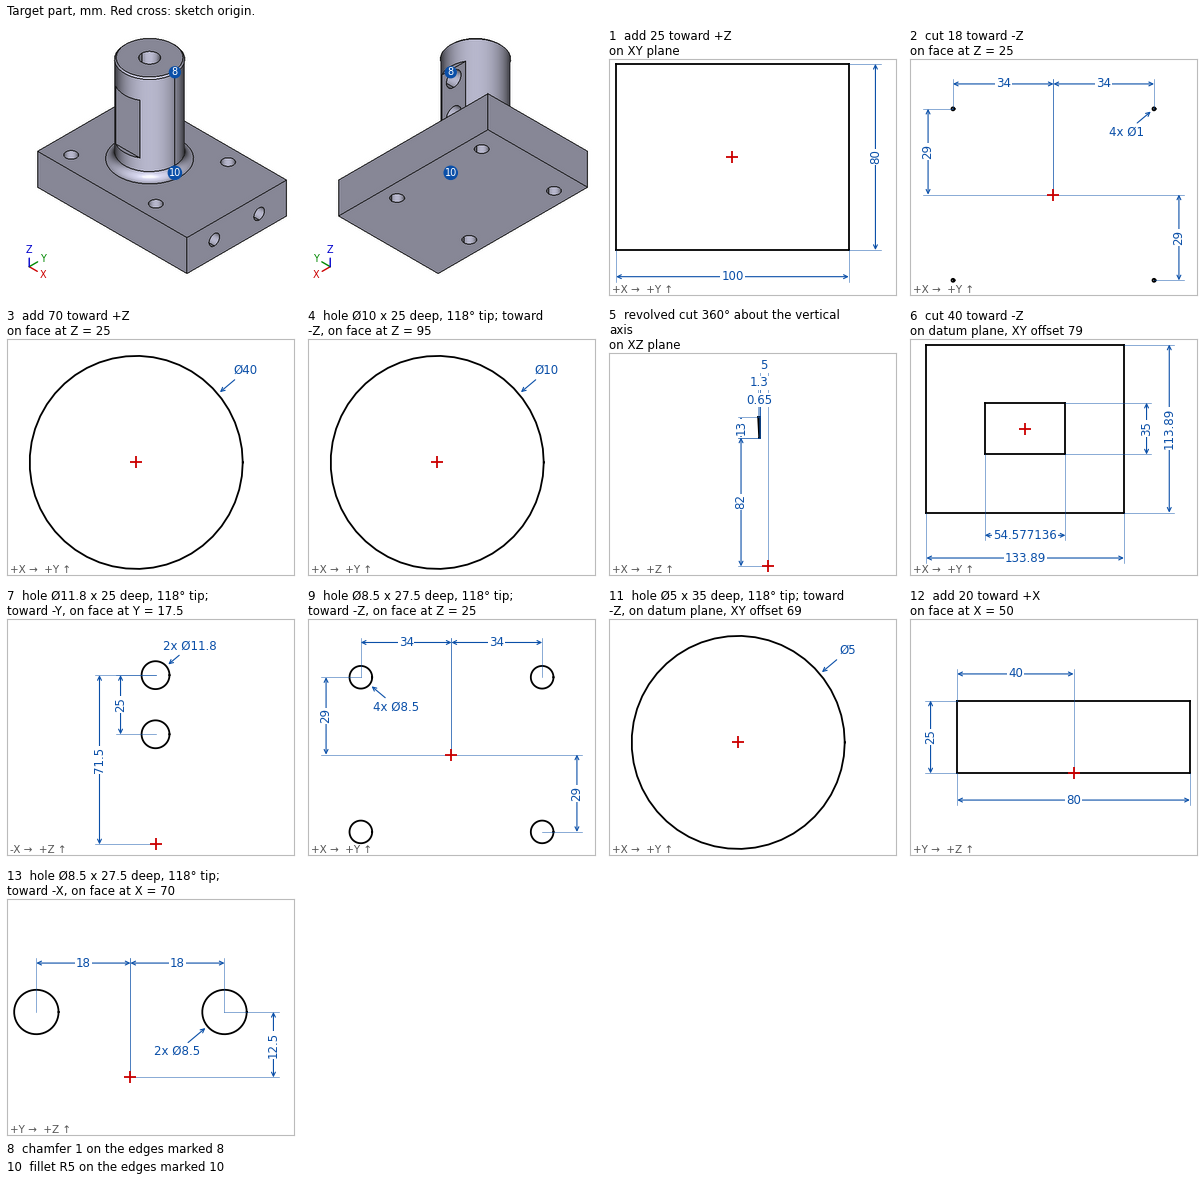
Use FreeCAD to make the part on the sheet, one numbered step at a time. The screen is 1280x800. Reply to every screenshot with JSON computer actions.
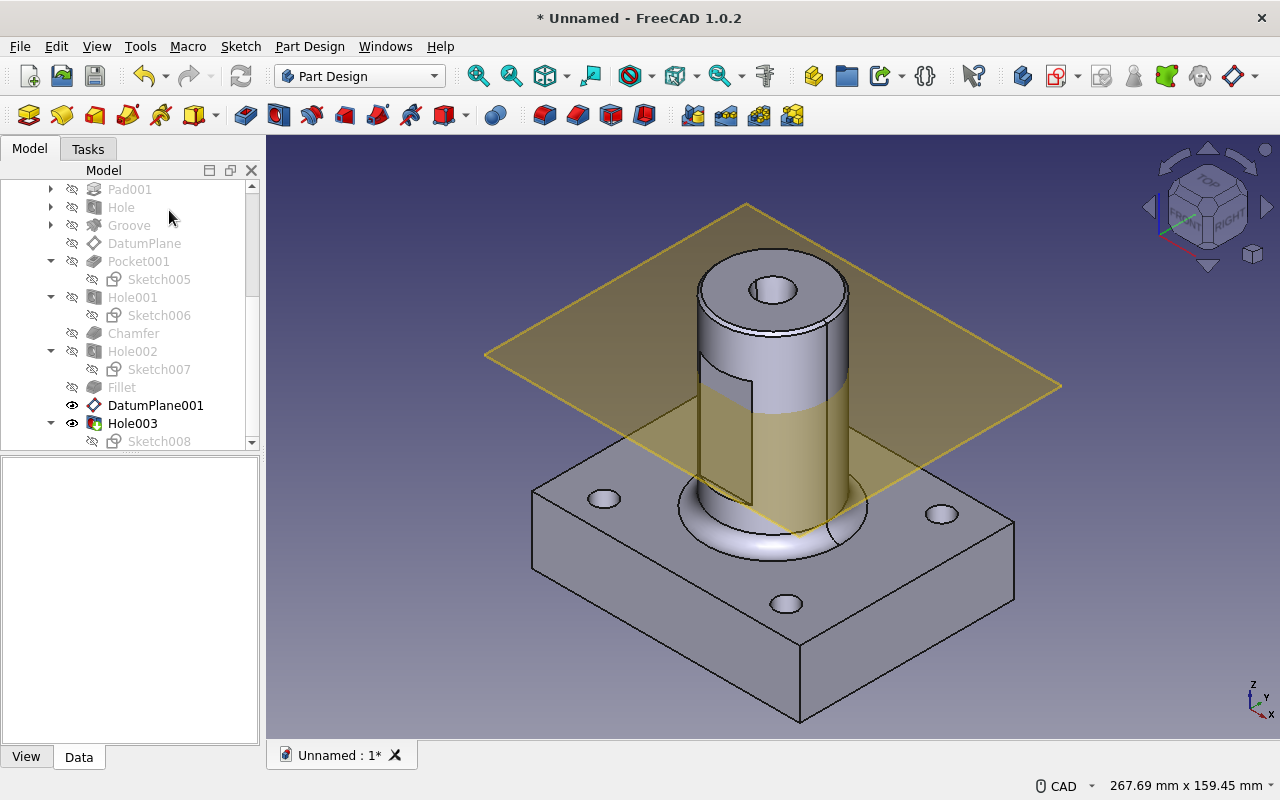
{"action": "left_click", "coordinate": [117, 405]}
{"action": "key", "text": "space"}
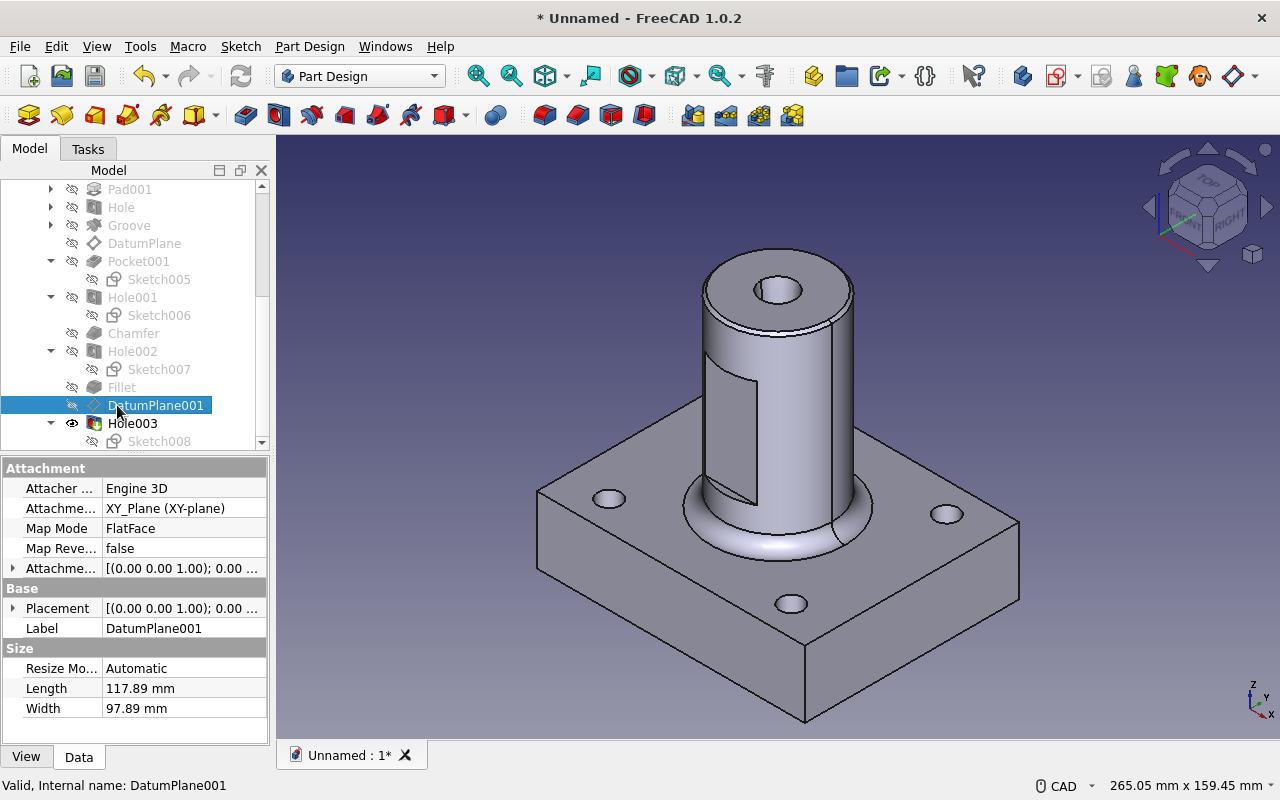
{"action": "left_click", "coordinate": [973, 586]}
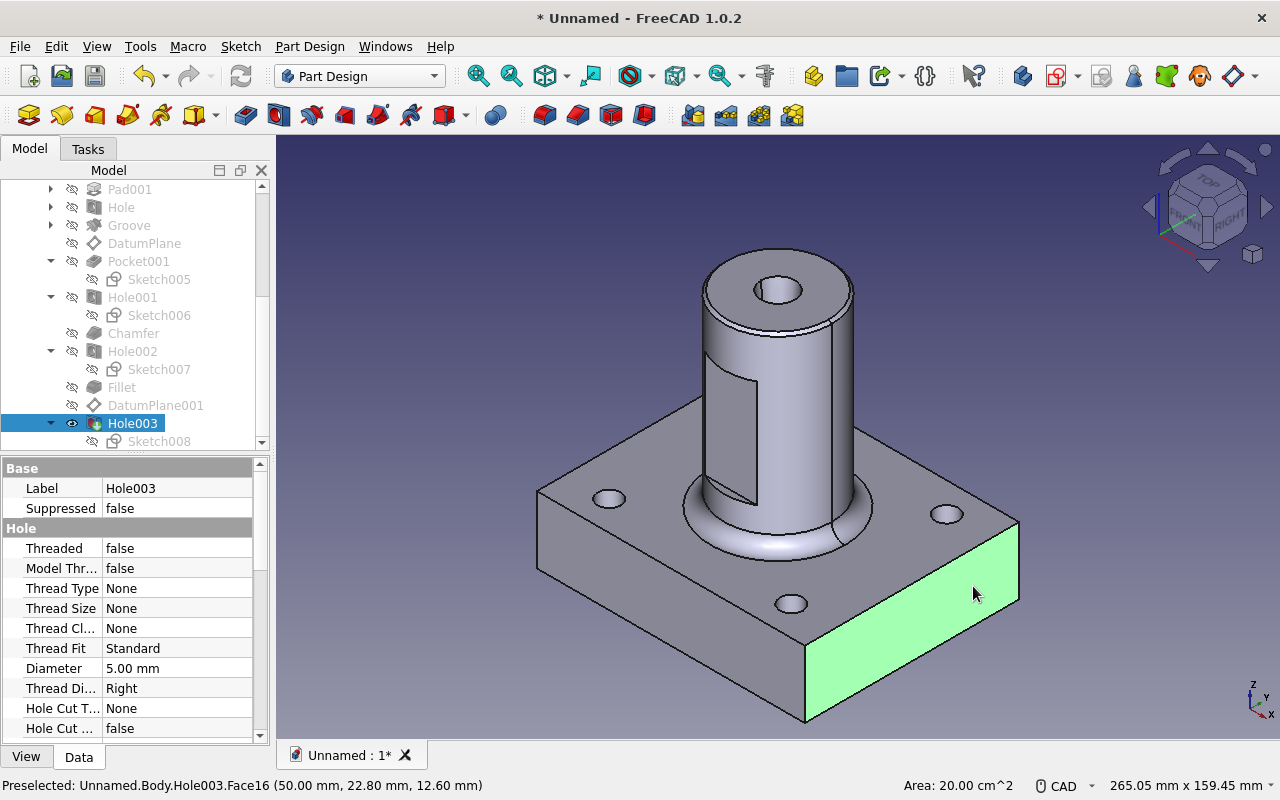
{"action": "left_click", "coordinate": [1056, 76]}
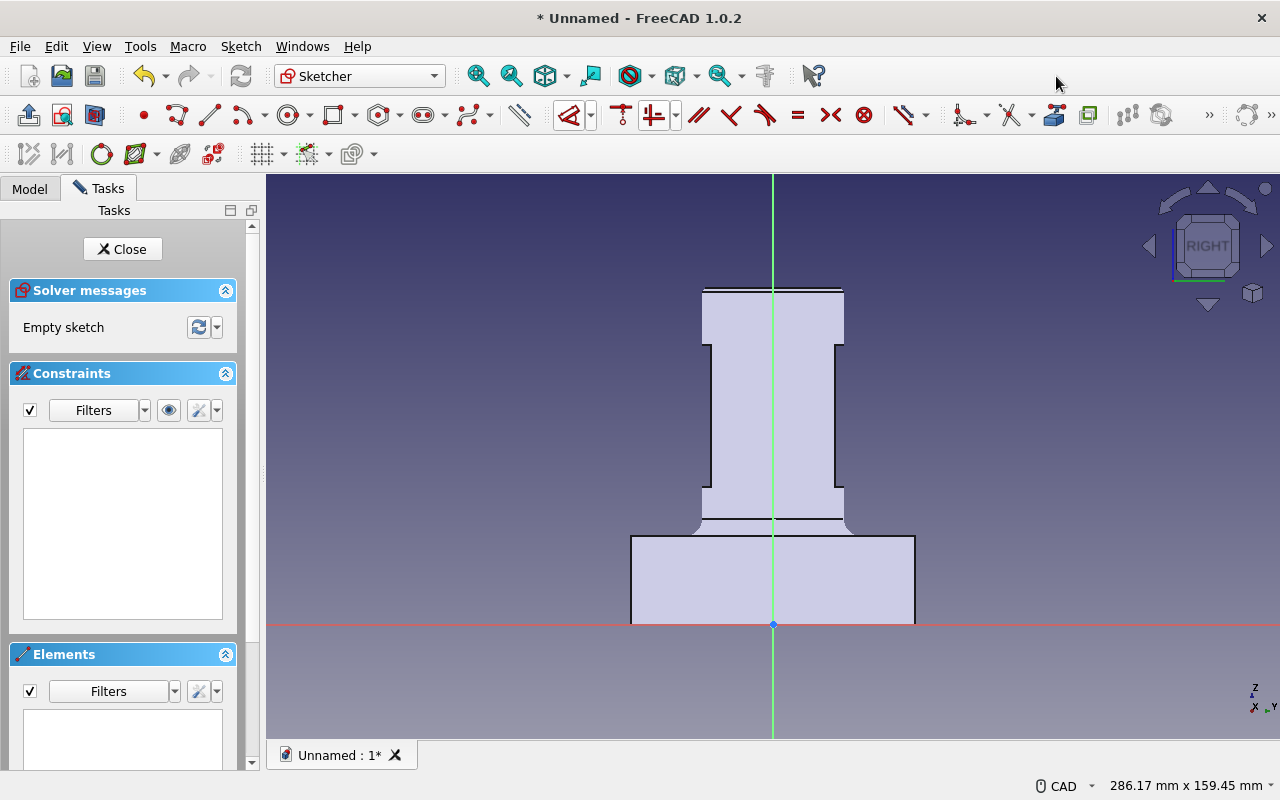
{"action": "scroll", "coordinate": [829, 682], "scroll_direction": "up", "scroll_amount": 4}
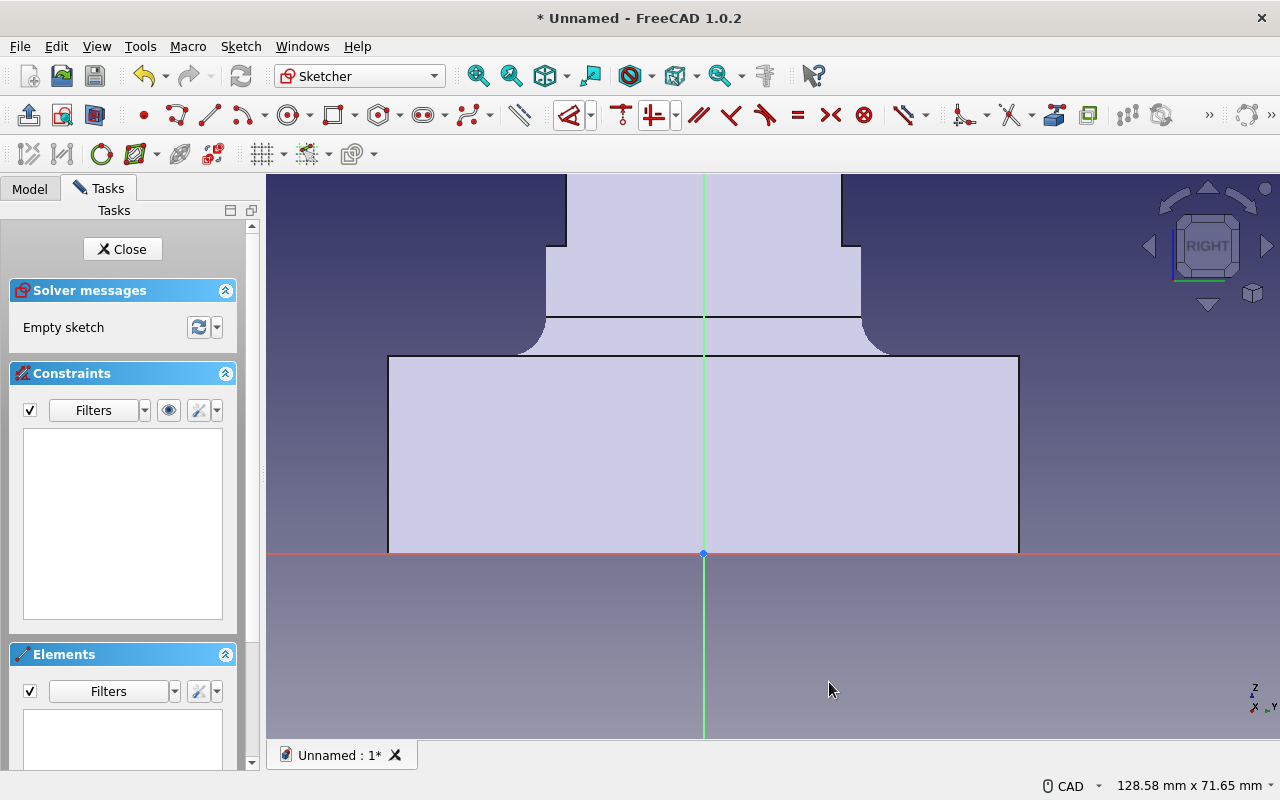
{"action": "key", "text": "g r"}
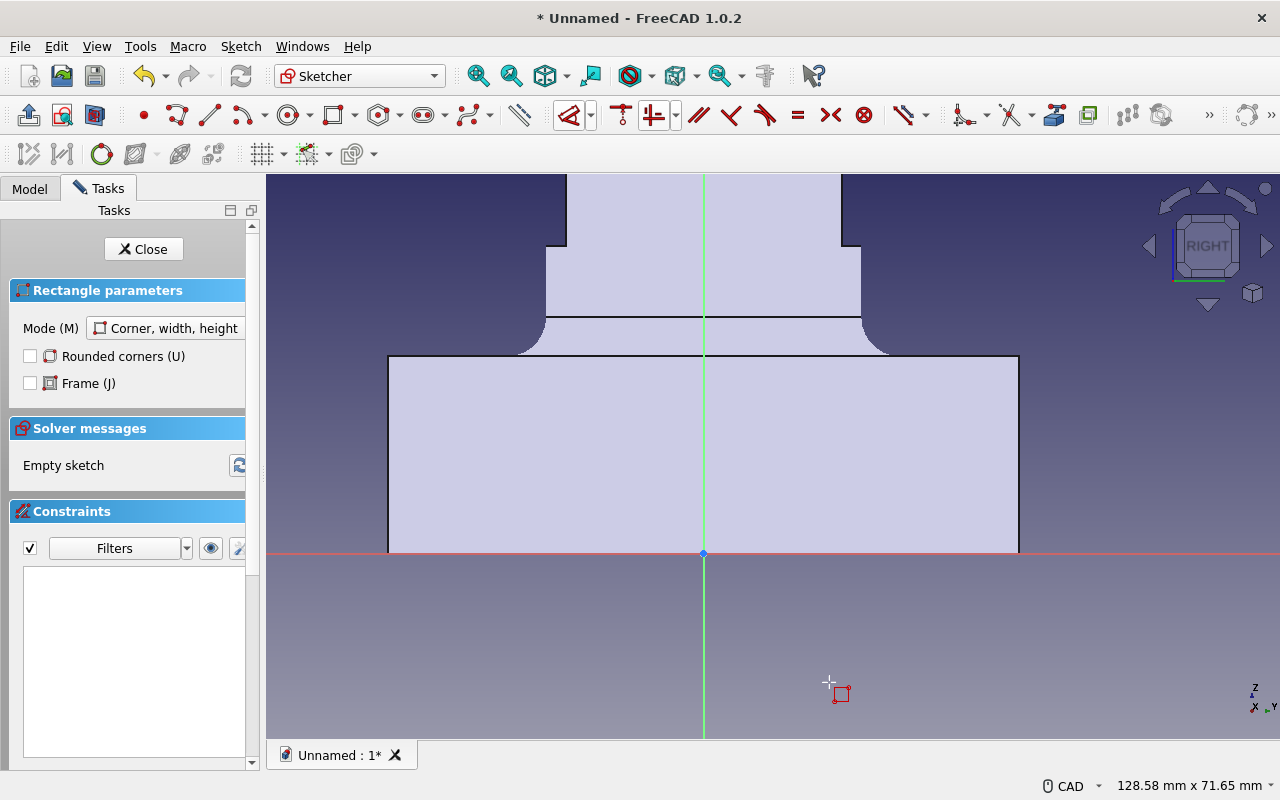
{"action": "left_click", "coordinate": [388, 356]}
{"action": "left_click", "coordinate": [1019, 554]}
{"action": "key", "text": "Escape"}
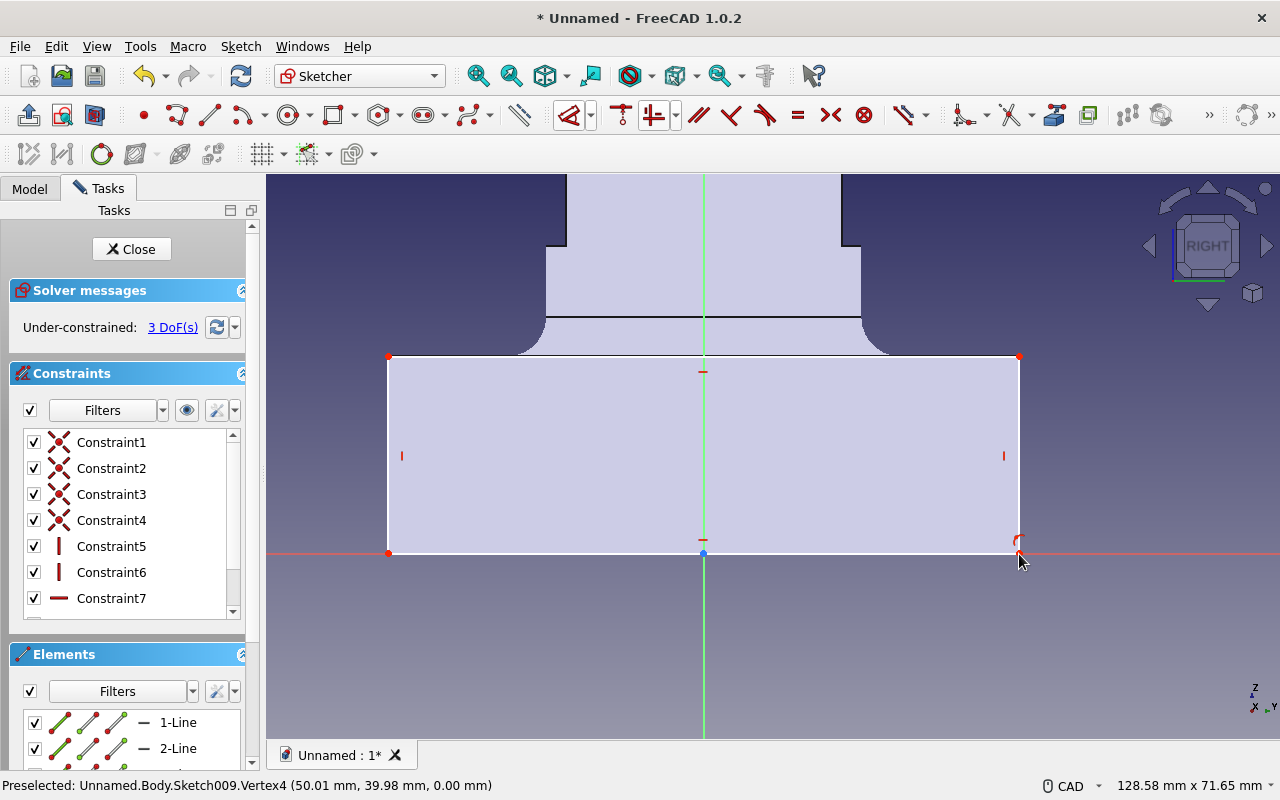
{"action": "left_click", "coordinate": [388, 416]}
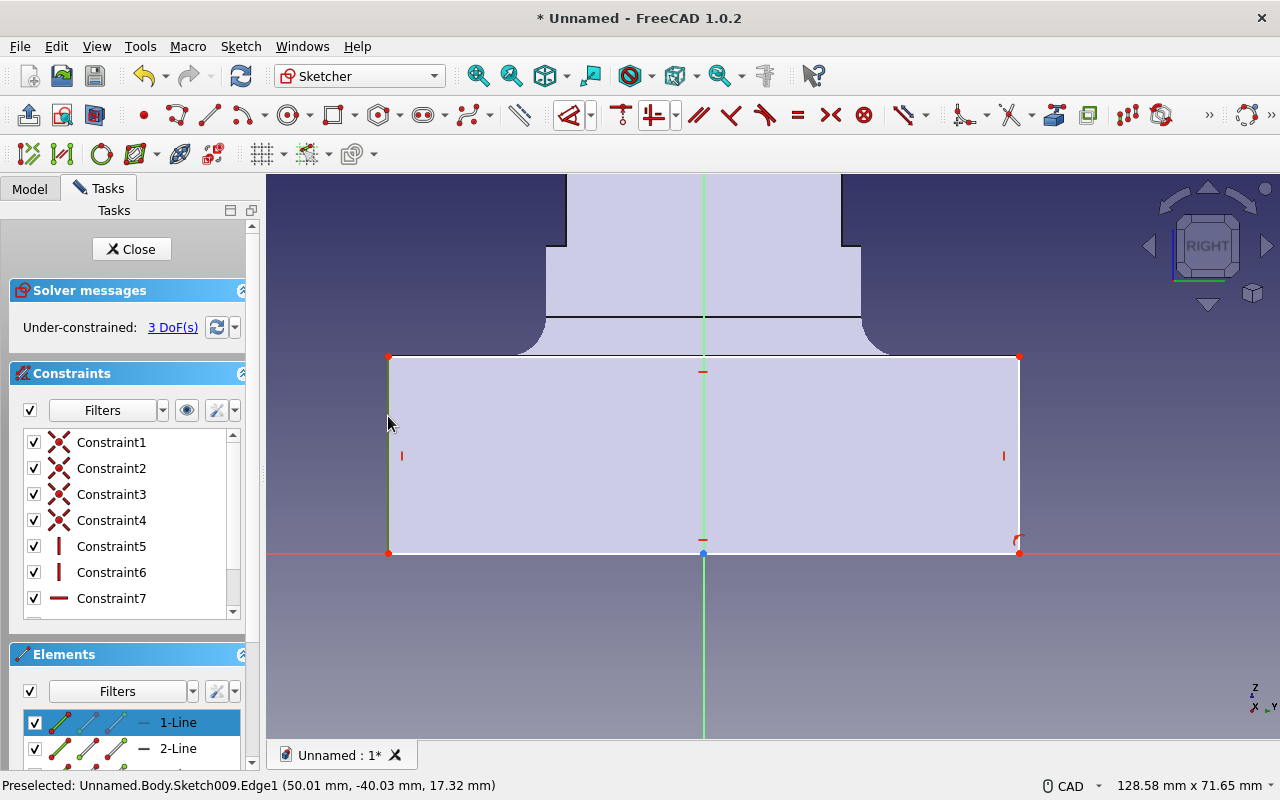
{"action": "key", "text": "i"}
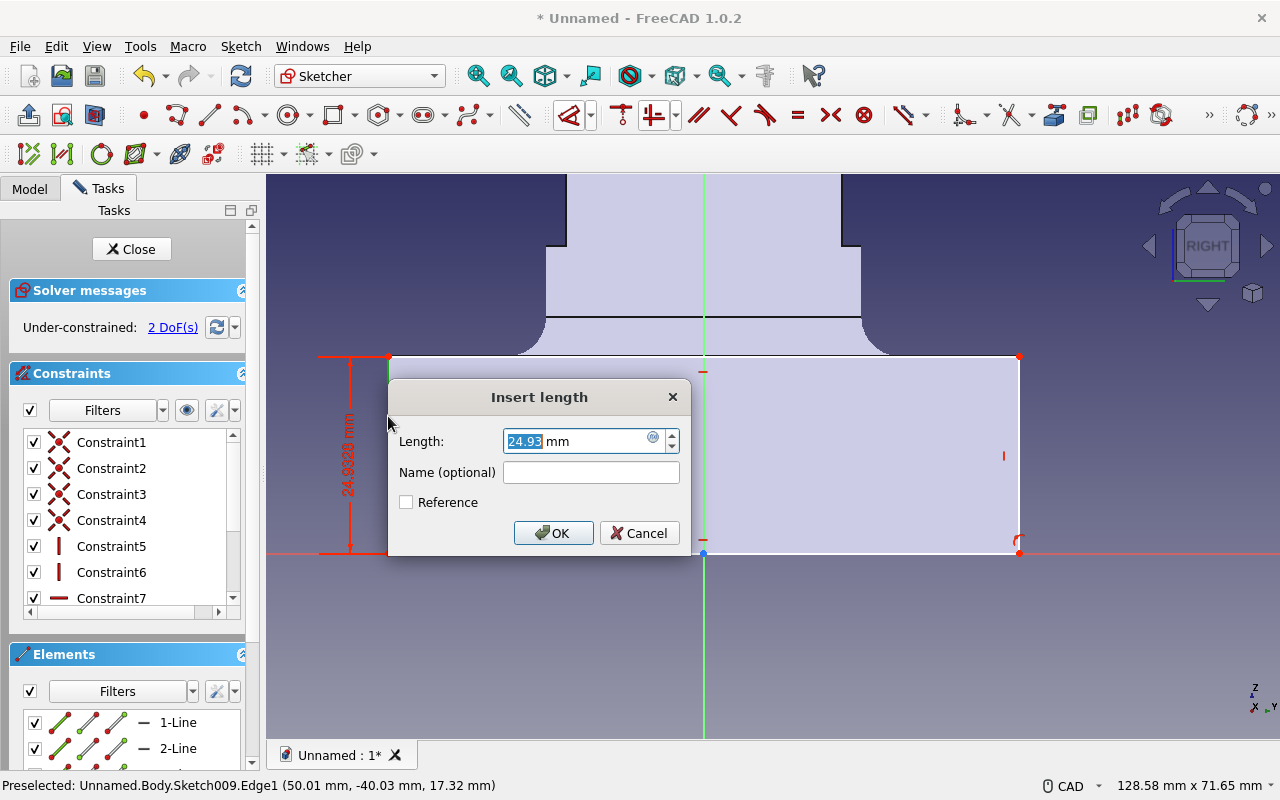
{"action": "type", "text": "25"}
{"action": "key", "text": "Return"}